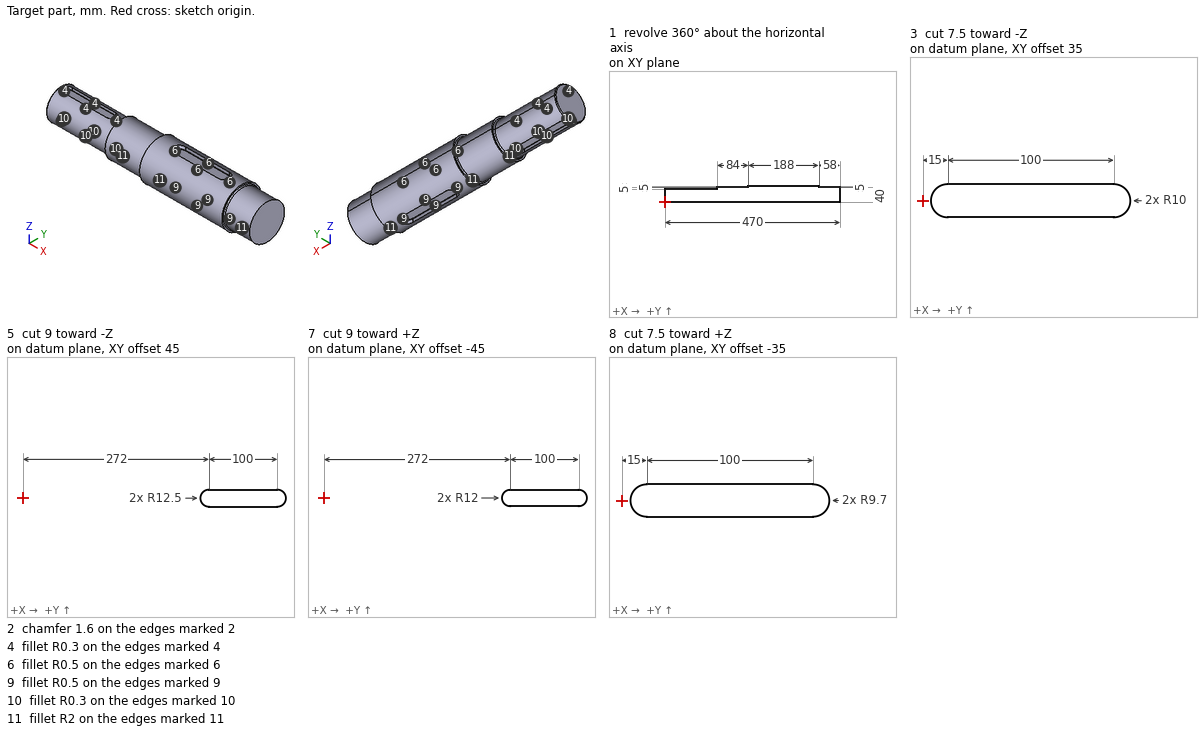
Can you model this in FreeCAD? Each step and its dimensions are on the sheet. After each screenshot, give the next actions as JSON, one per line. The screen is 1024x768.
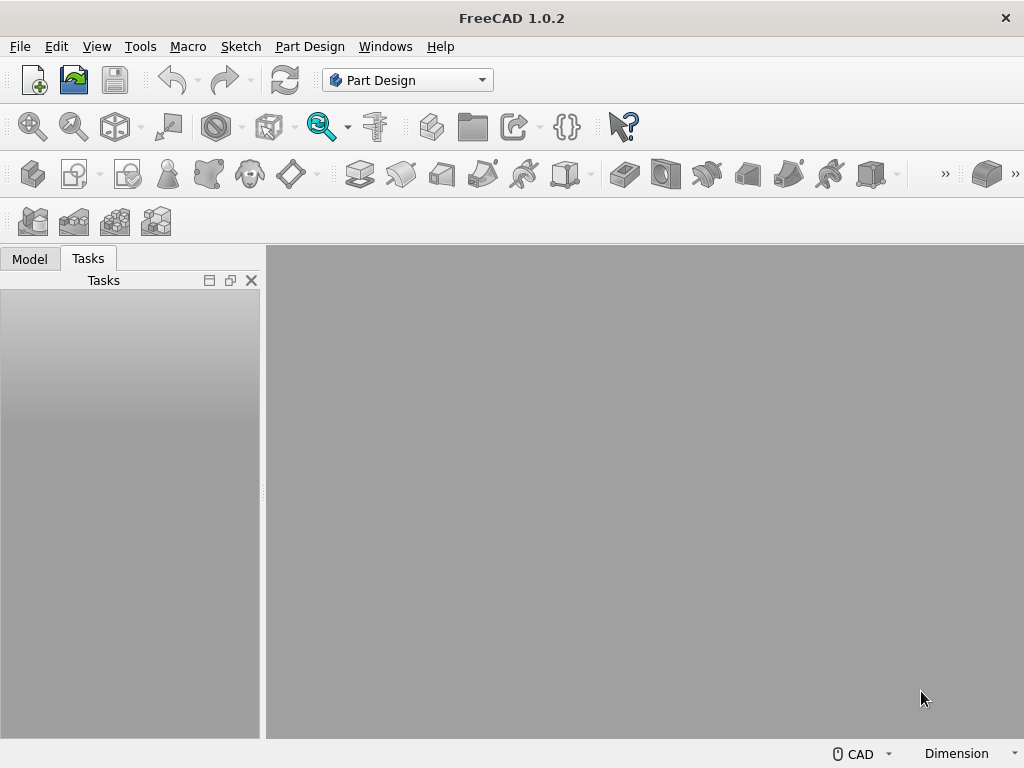
{"action": "left_click", "coordinate": [33, 80]}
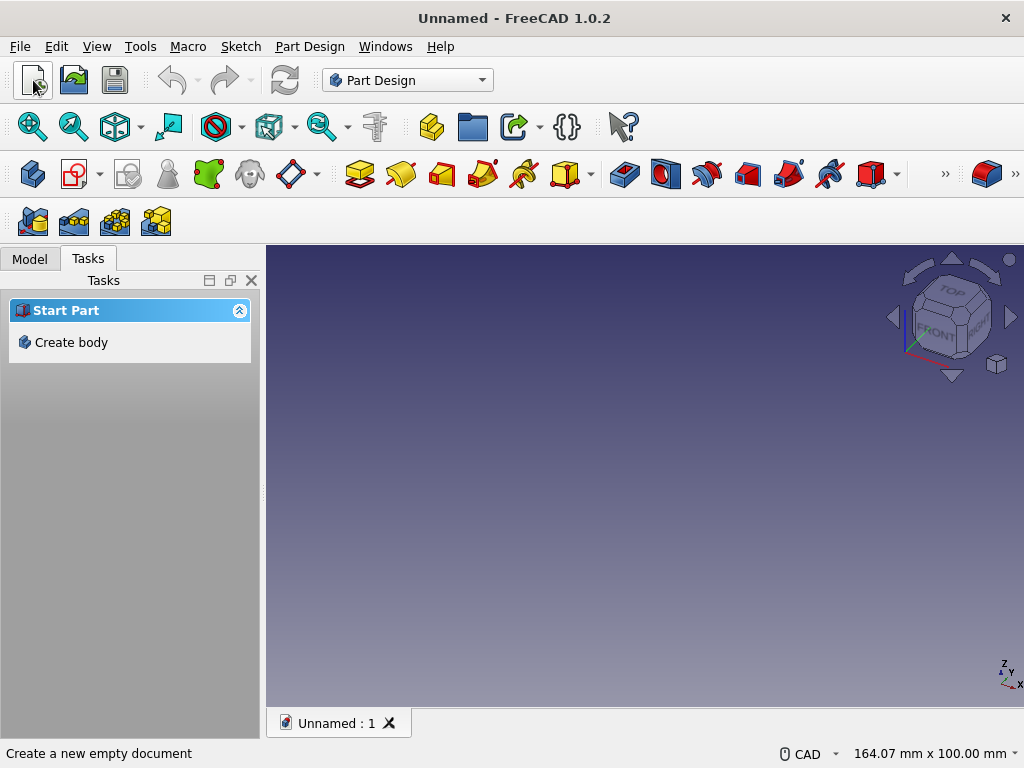
{"action": "left_click", "coordinate": [74, 174]}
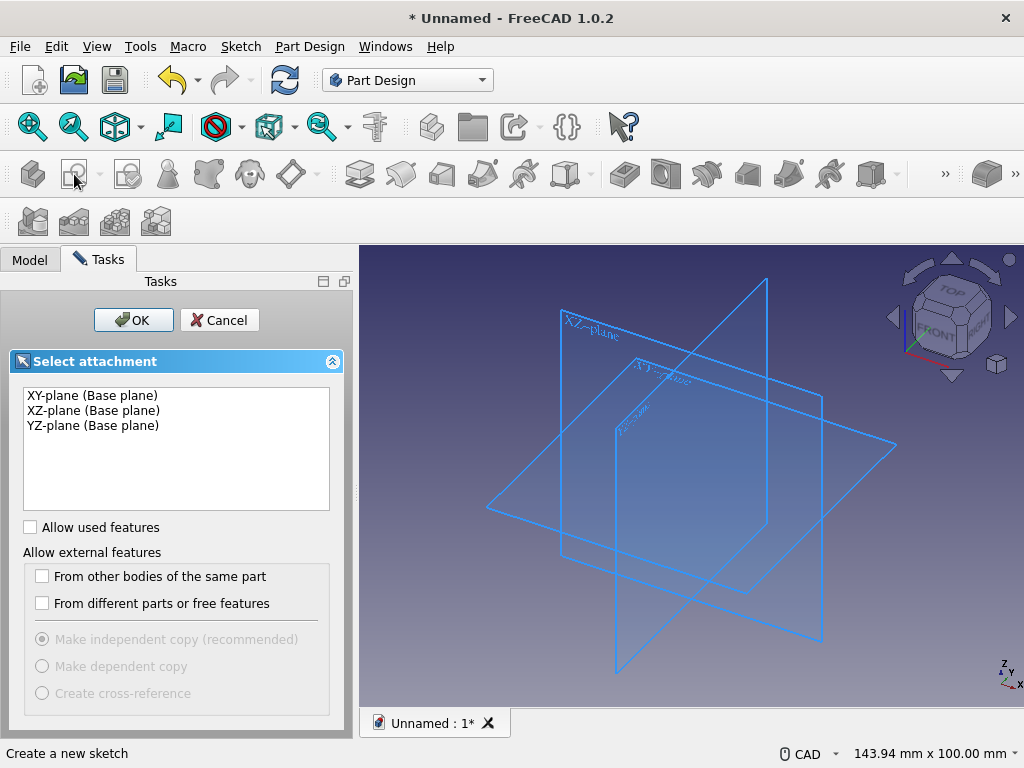
{"action": "left_click", "coordinate": [84, 396]}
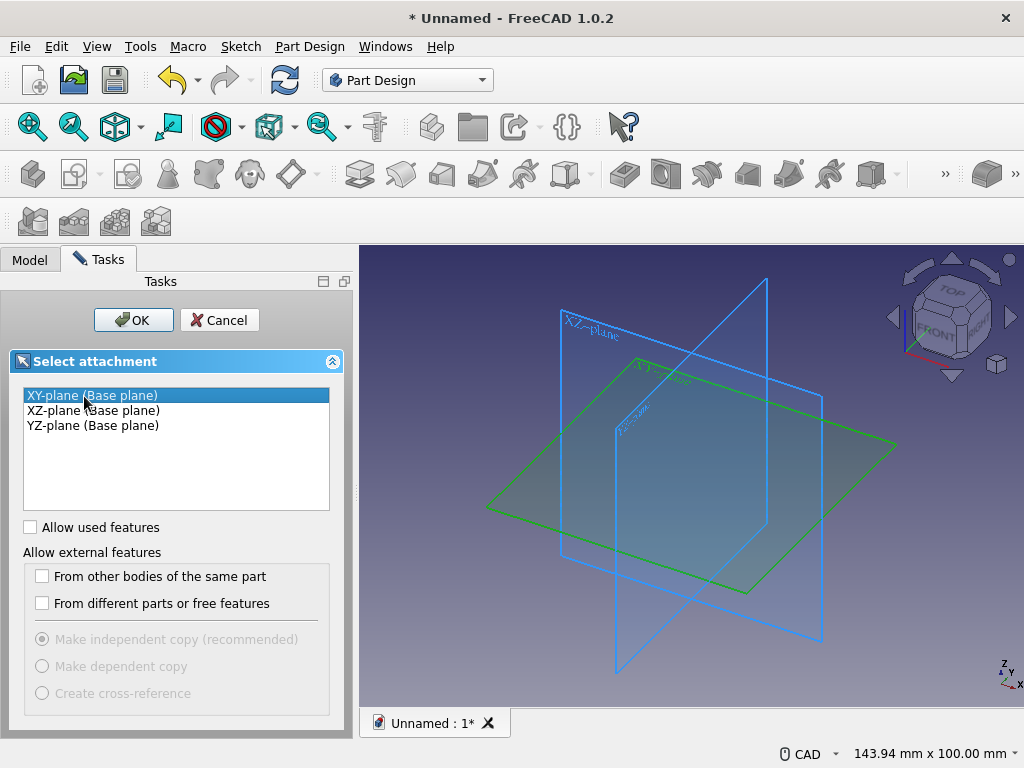
{"action": "left_click", "coordinate": [134, 320]}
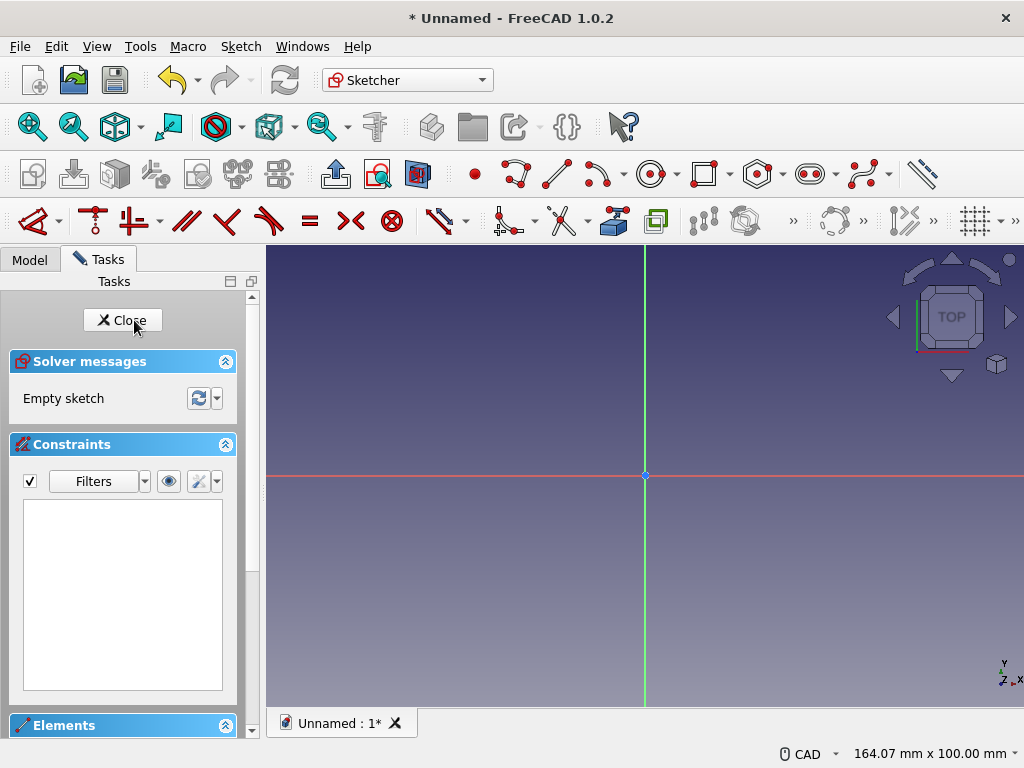
{"action": "scroll", "coordinate": [294, 502], "scroll_direction": "down", "scroll_amount": 8}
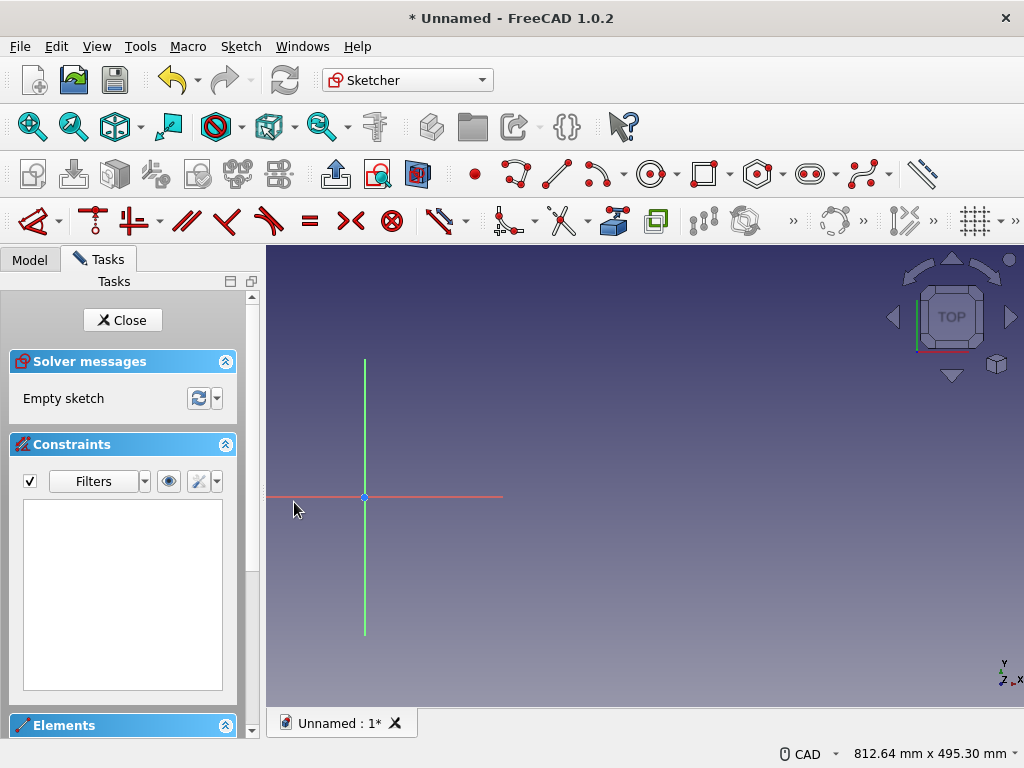
{"action": "left_click", "coordinate": [516, 174]}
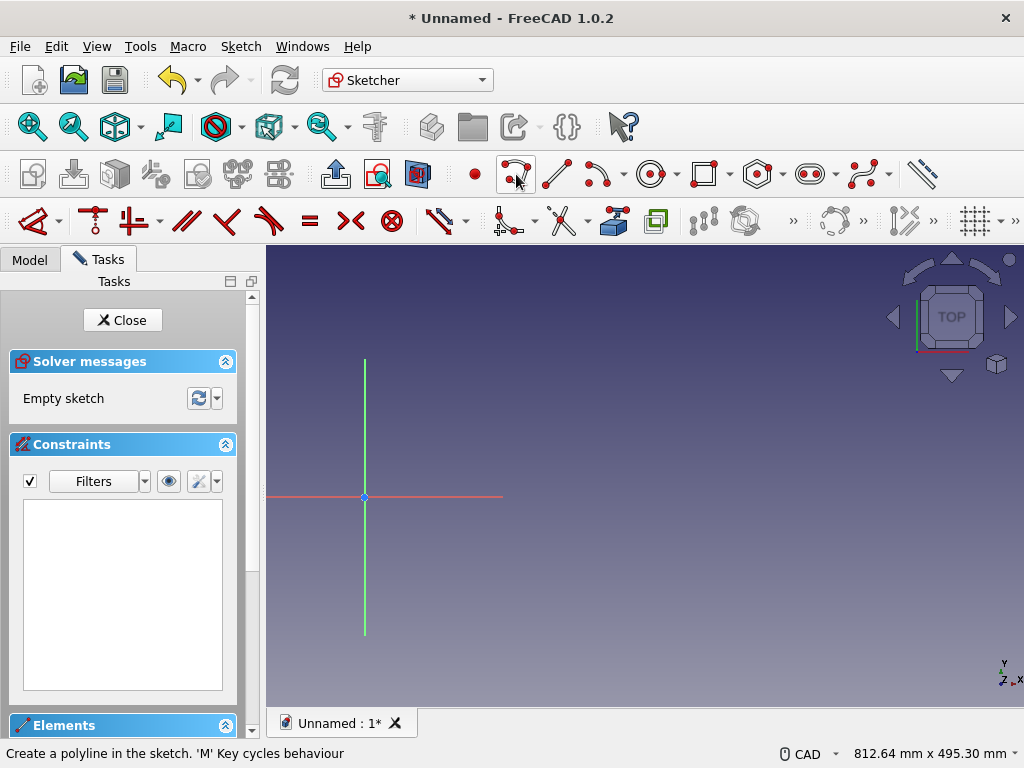
{"action": "left_click", "coordinate": [365, 497]}
{"action": "left_click", "coordinate": [803, 488]}
{"action": "left_click", "coordinate": [803, 460]}
{"action": "left_click", "coordinate": [749, 460]}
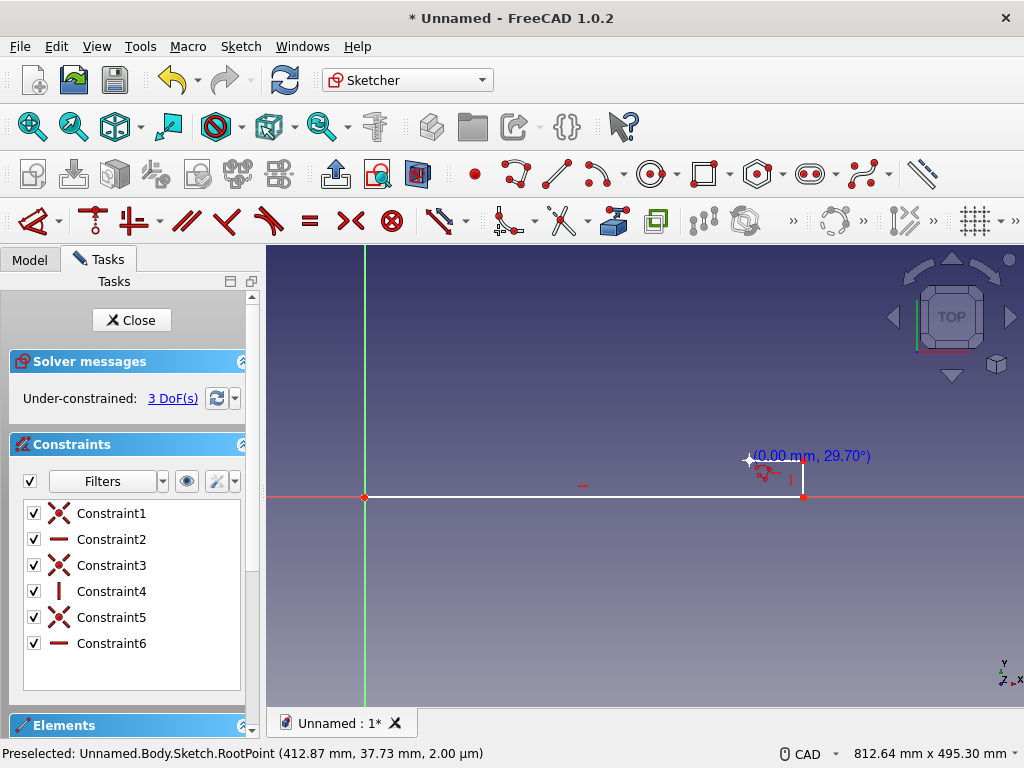
{"action": "scroll", "coordinate": [749, 455], "scroll_direction": "up", "scroll_amount": 7}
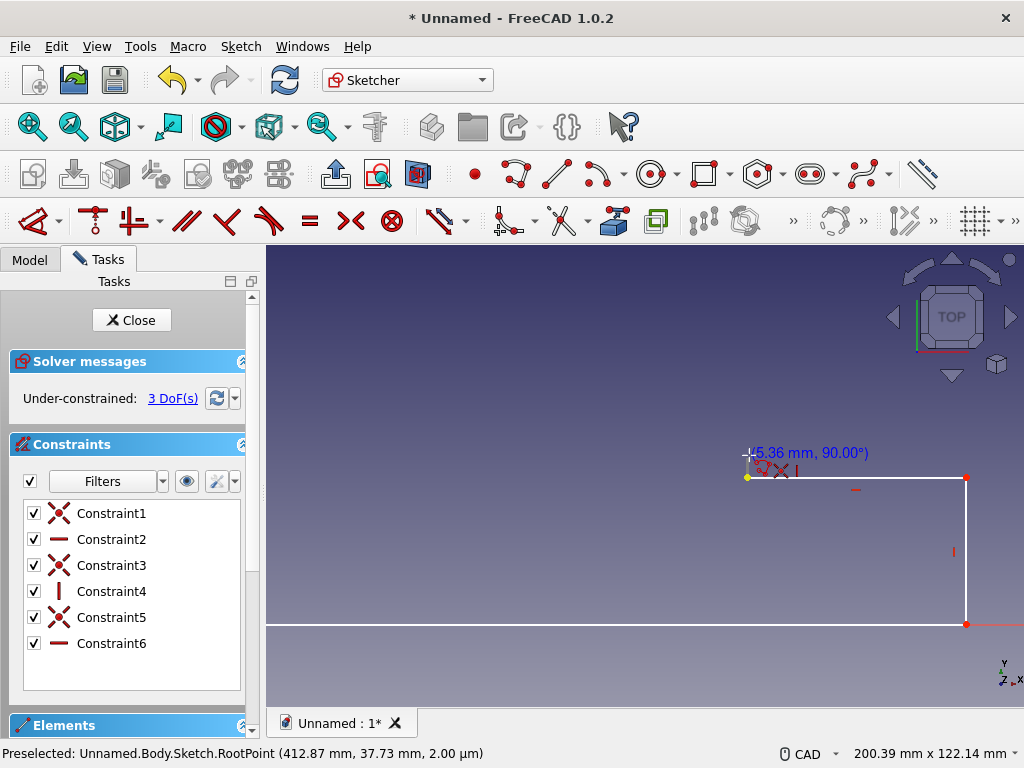
{"action": "left_click", "coordinate": [747, 455]}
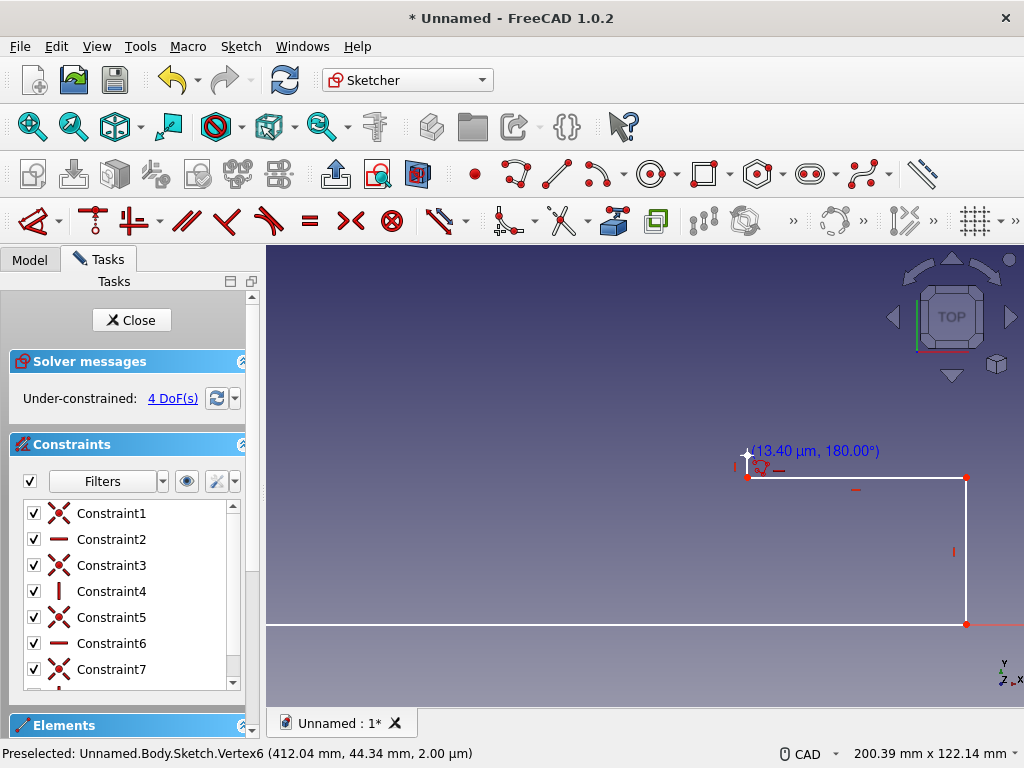
{"action": "scroll", "coordinate": [740, 455], "scroll_direction": "down", "scroll_amount": 7}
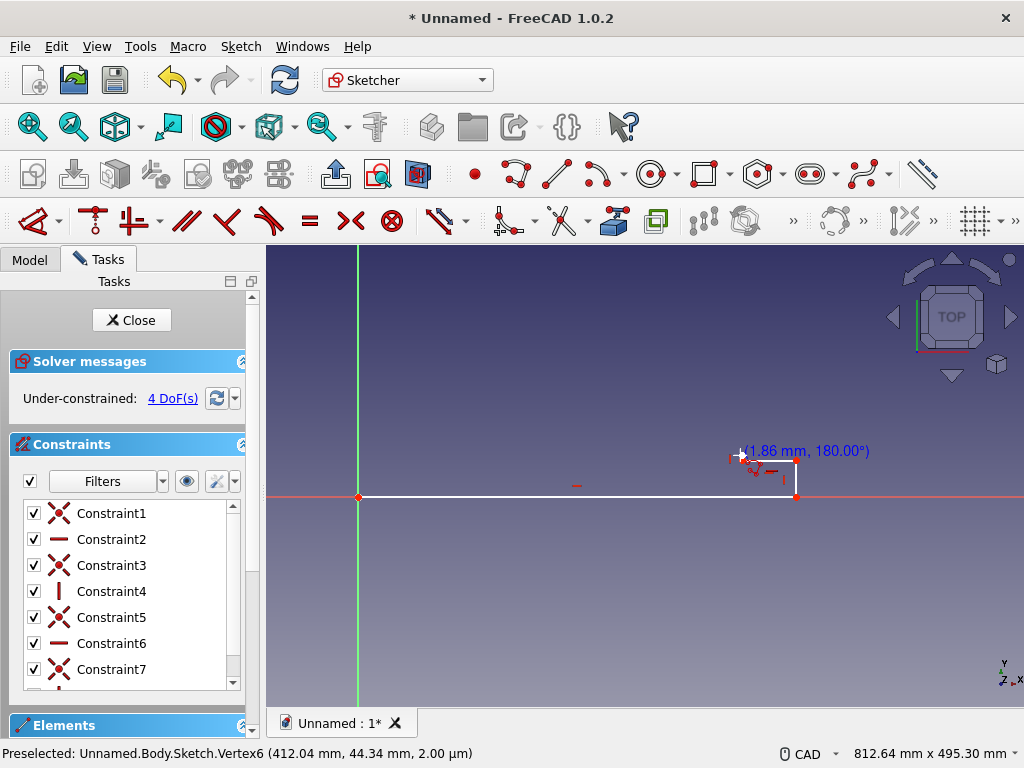
{"action": "left_click", "coordinate": [567, 455]}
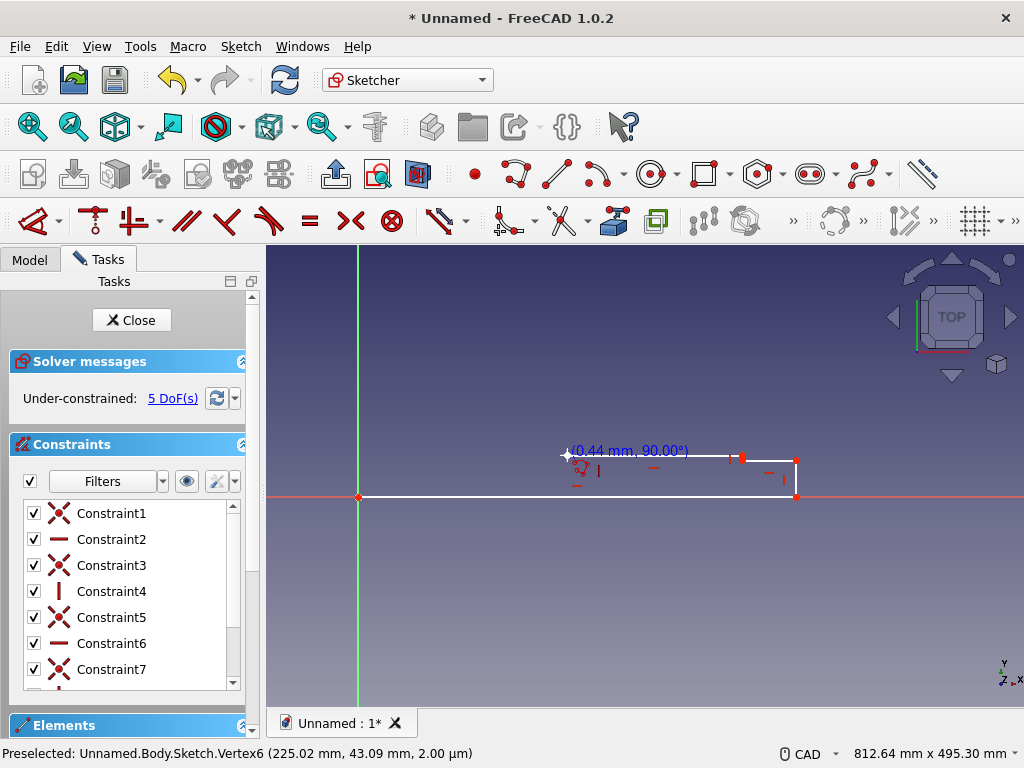
{"action": "scroll", "coordinate": [567, 460], "scroll_direction": "up", "scroll_amount": 7}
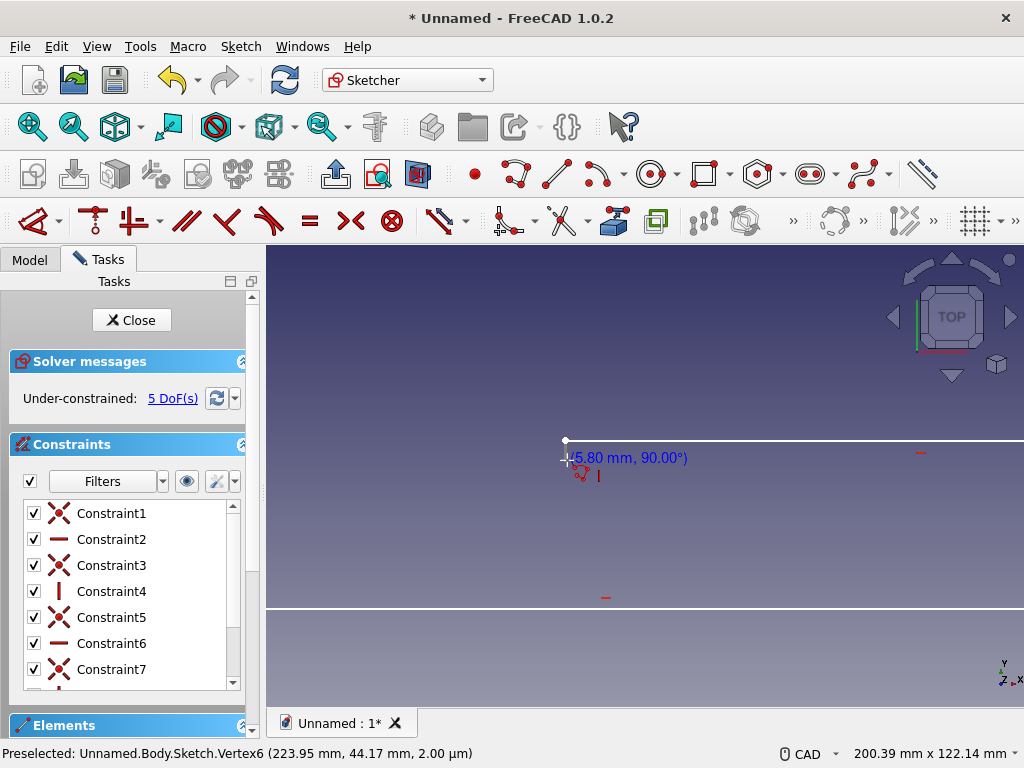
{"action": "left_click", "coordinate": [566, 458]}